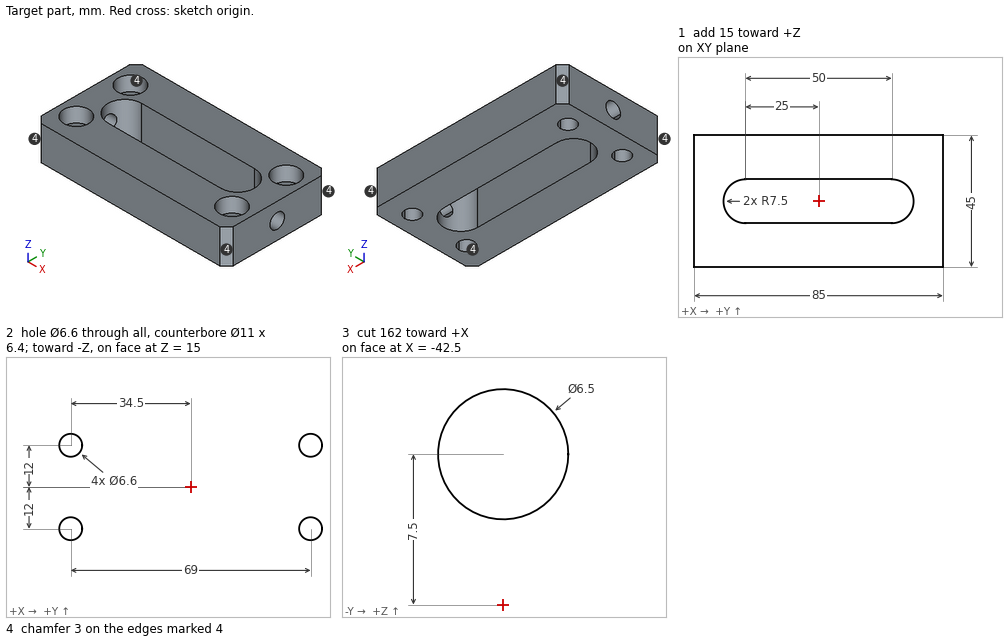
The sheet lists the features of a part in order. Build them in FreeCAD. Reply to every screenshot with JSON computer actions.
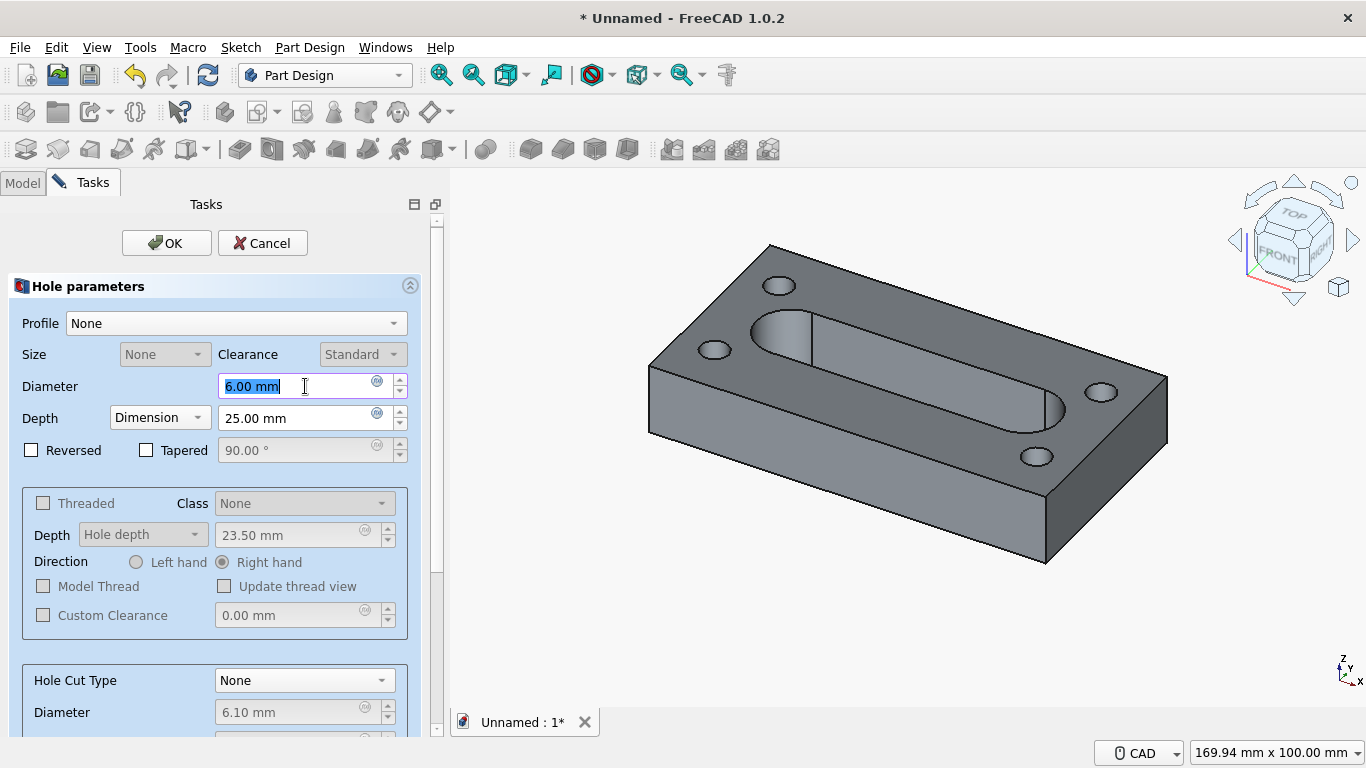
{"action": "type", "text": "6.6"}
{"action": "key", "text": "Tab"}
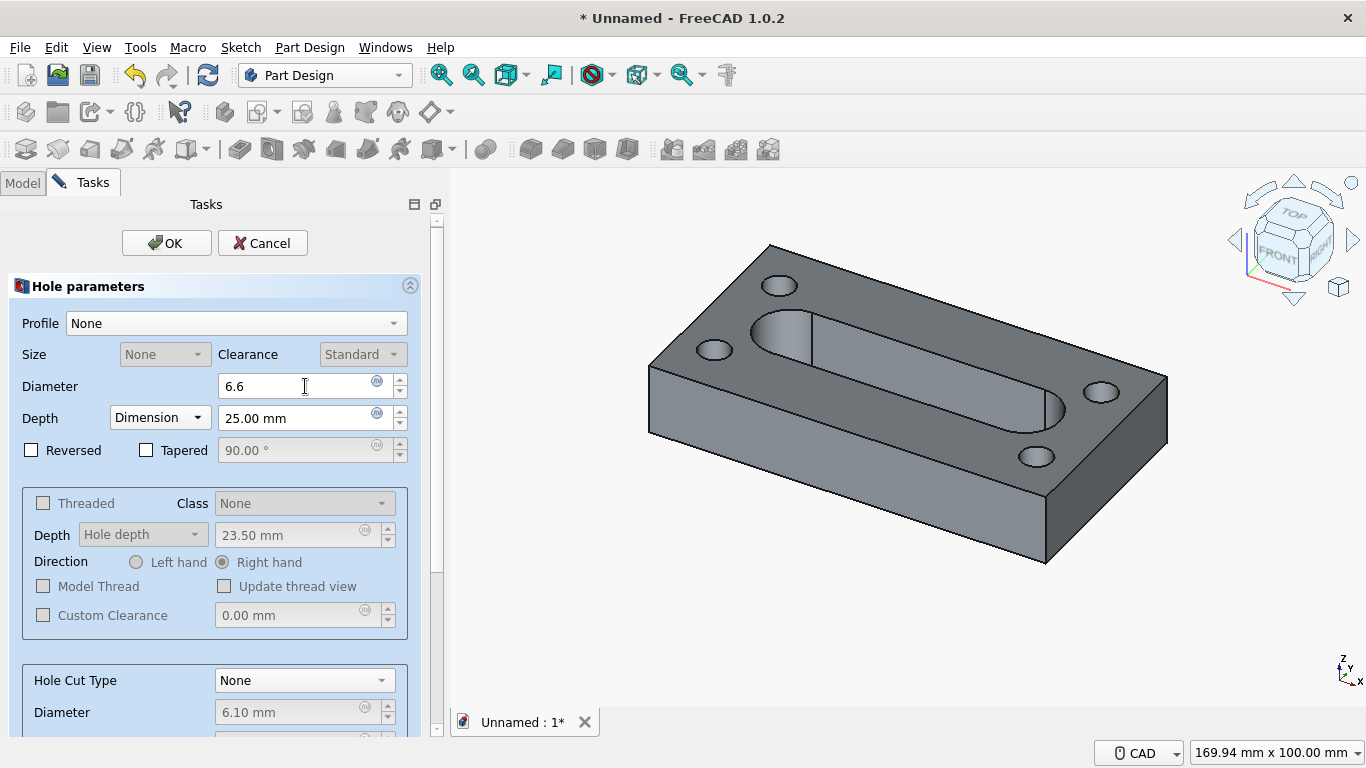
{"action": "left_click", "coordinate": [161, 418]}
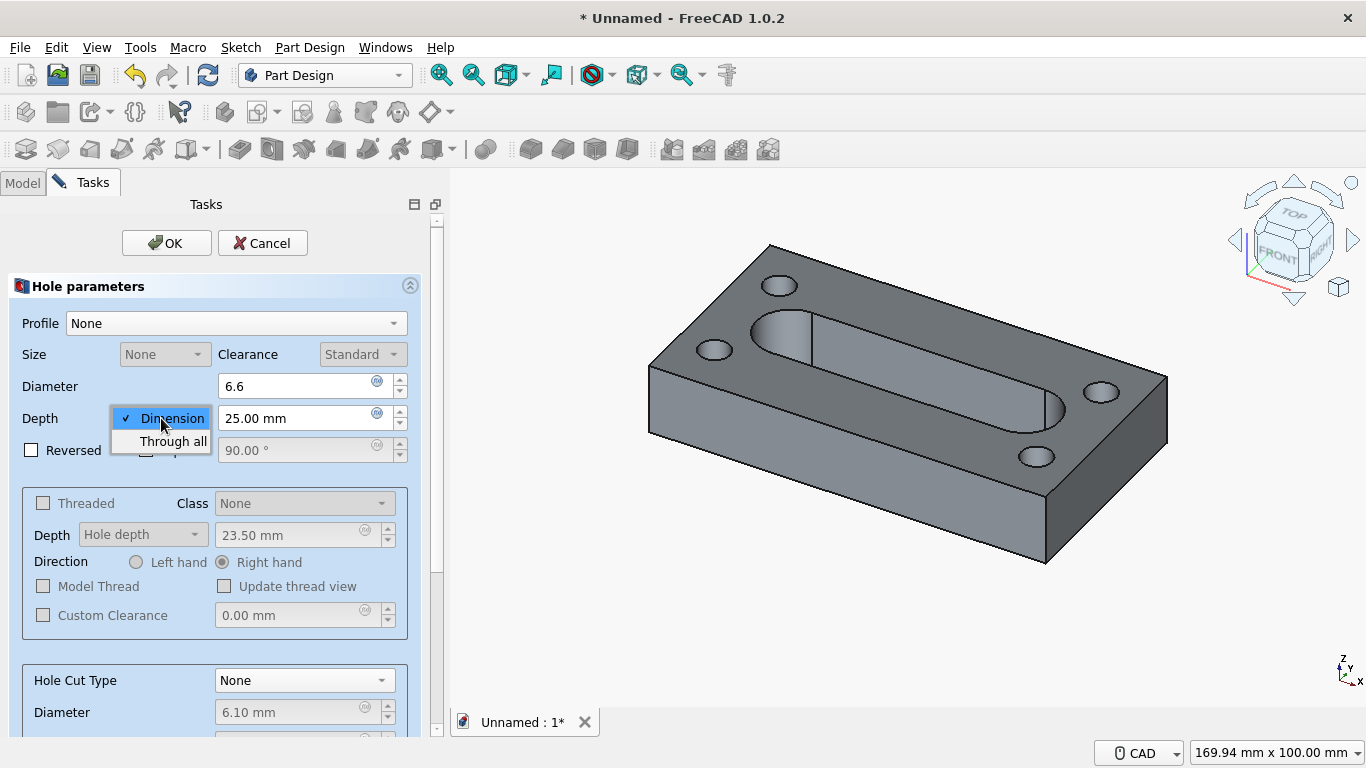
{"action": "left_click", "coordinate": [160, 442]}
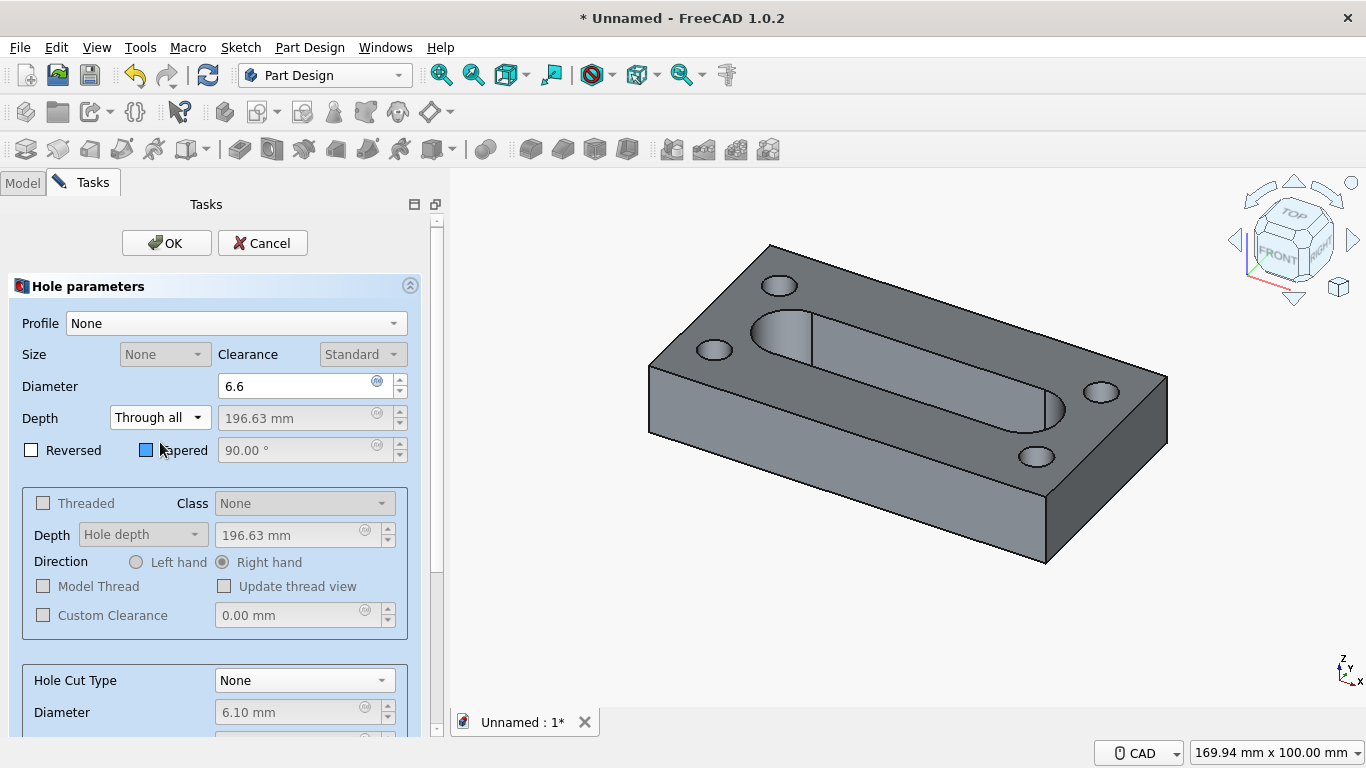
{"action": "left_click", "coordinate": [306, 680]}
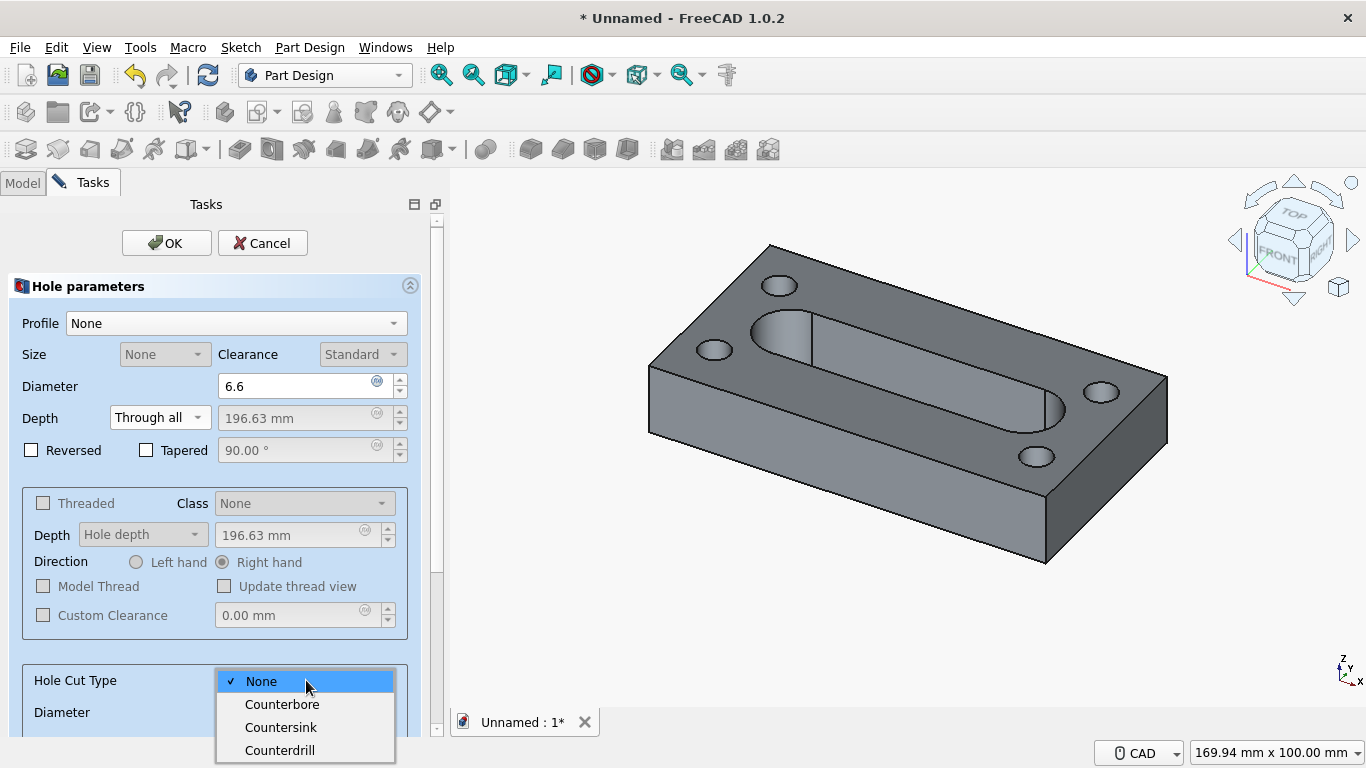
{"action": "left_click", "coordinate": [304, 704]}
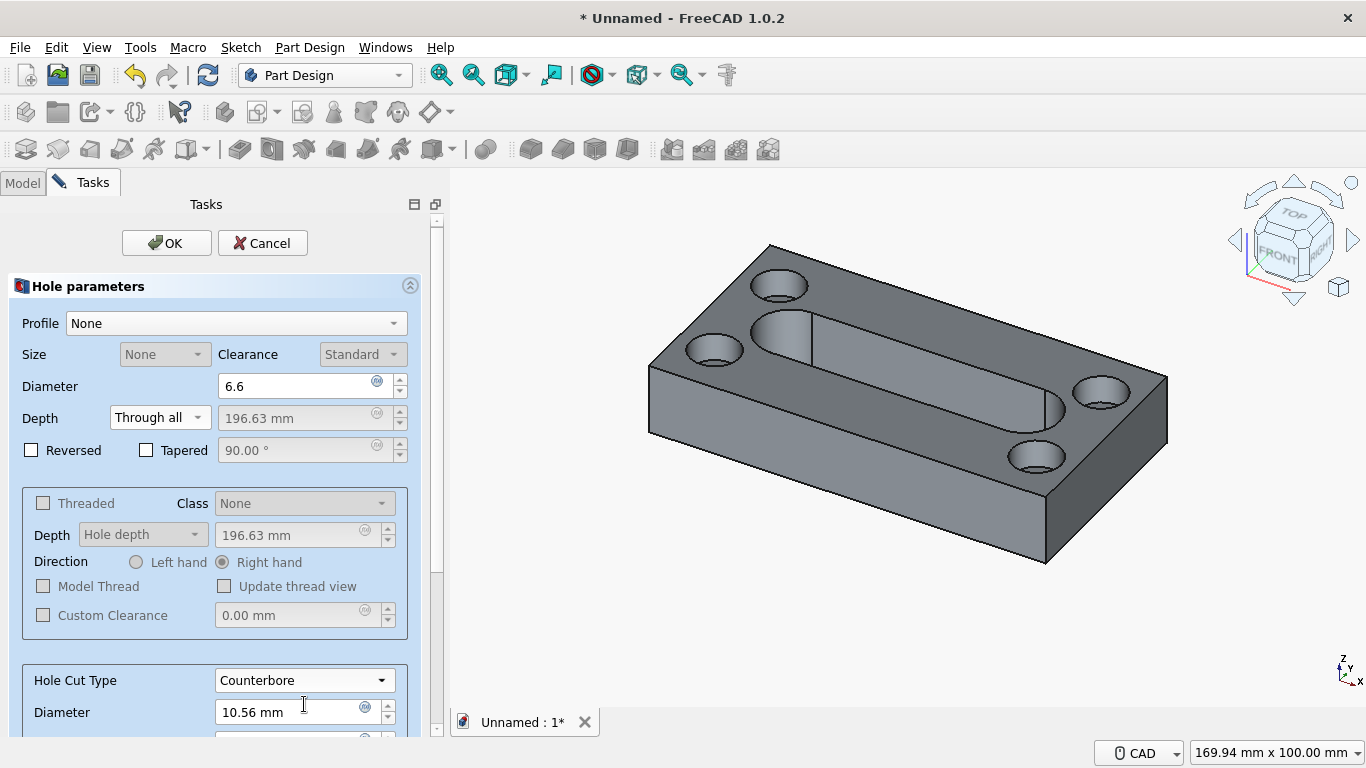
{"action": "triple_click", "coordinate": [298, 712]}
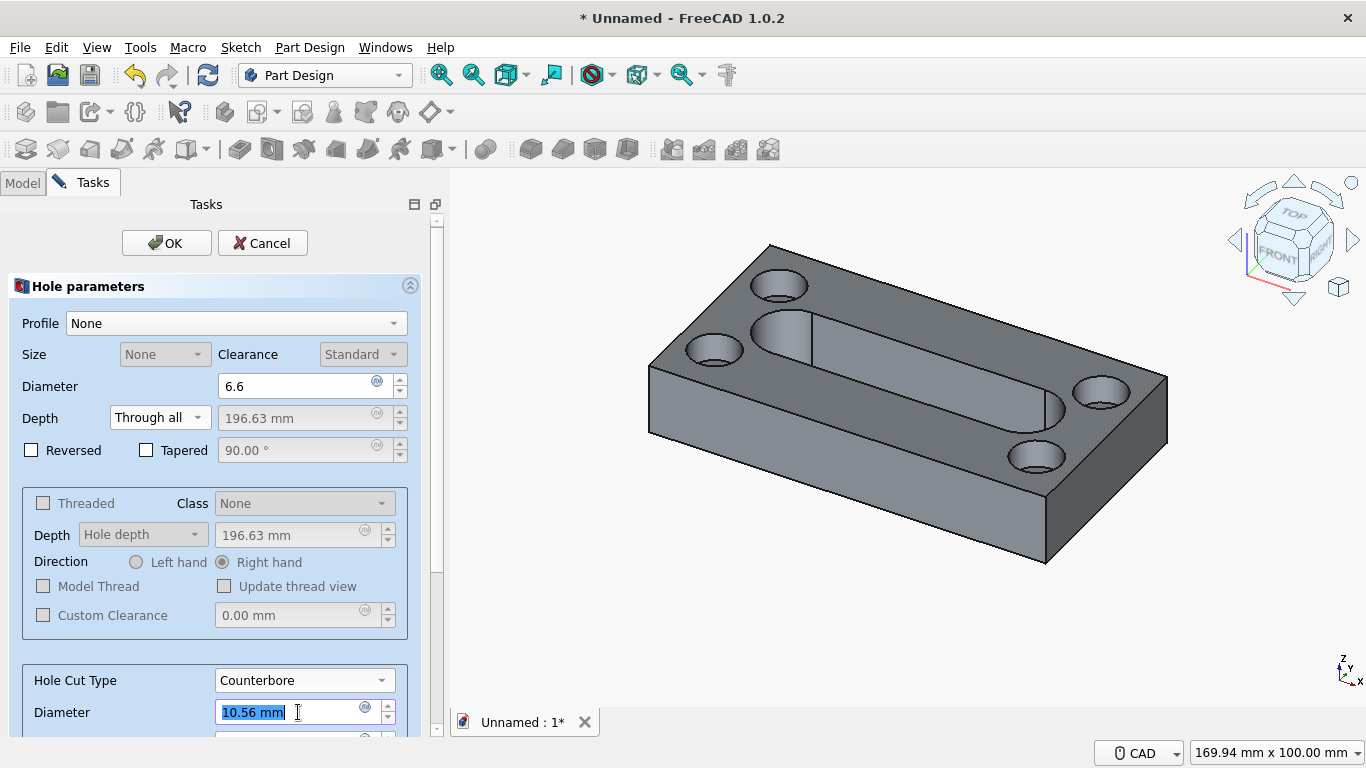
{"action": "type", "text": "11"}
{"action": "key", "text": "Tab"}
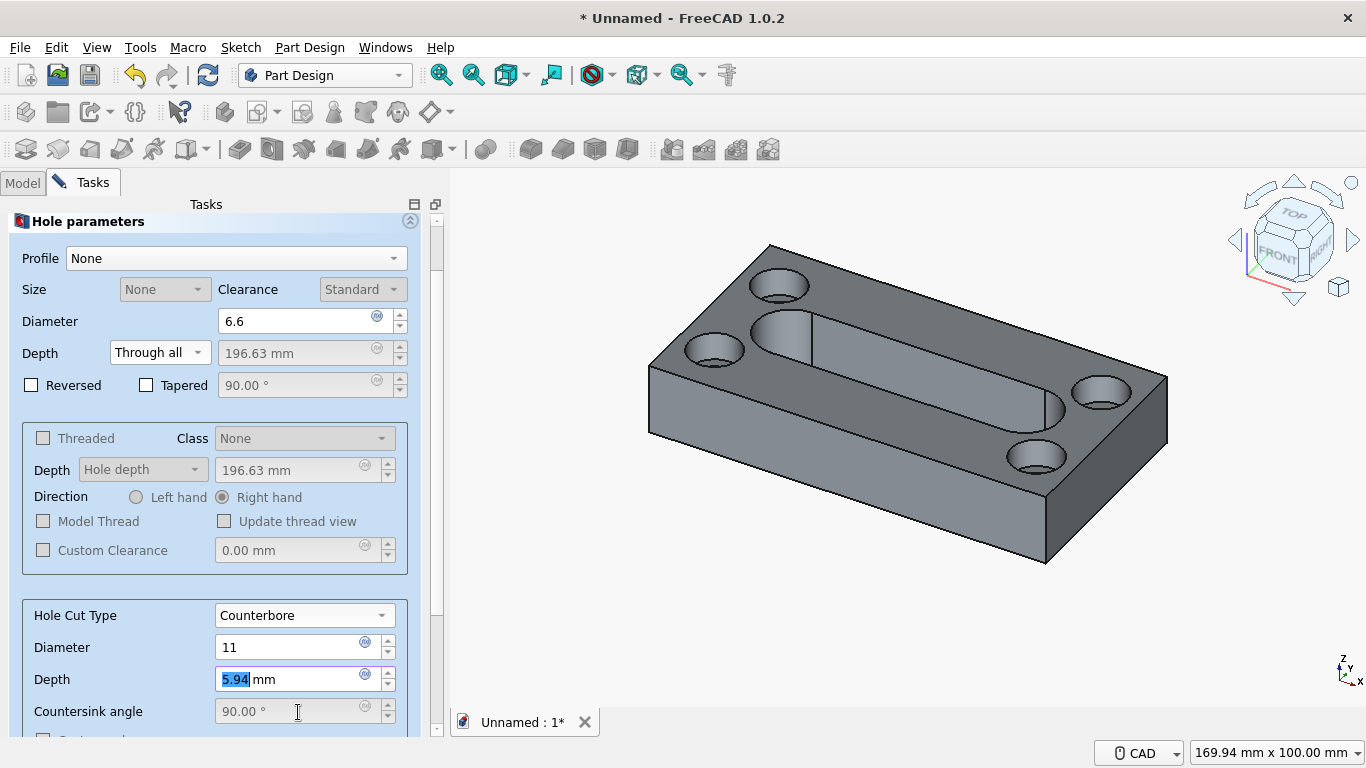
{"action": "type", "text": "6.4"}
{"action": "key", "text": "Tab"}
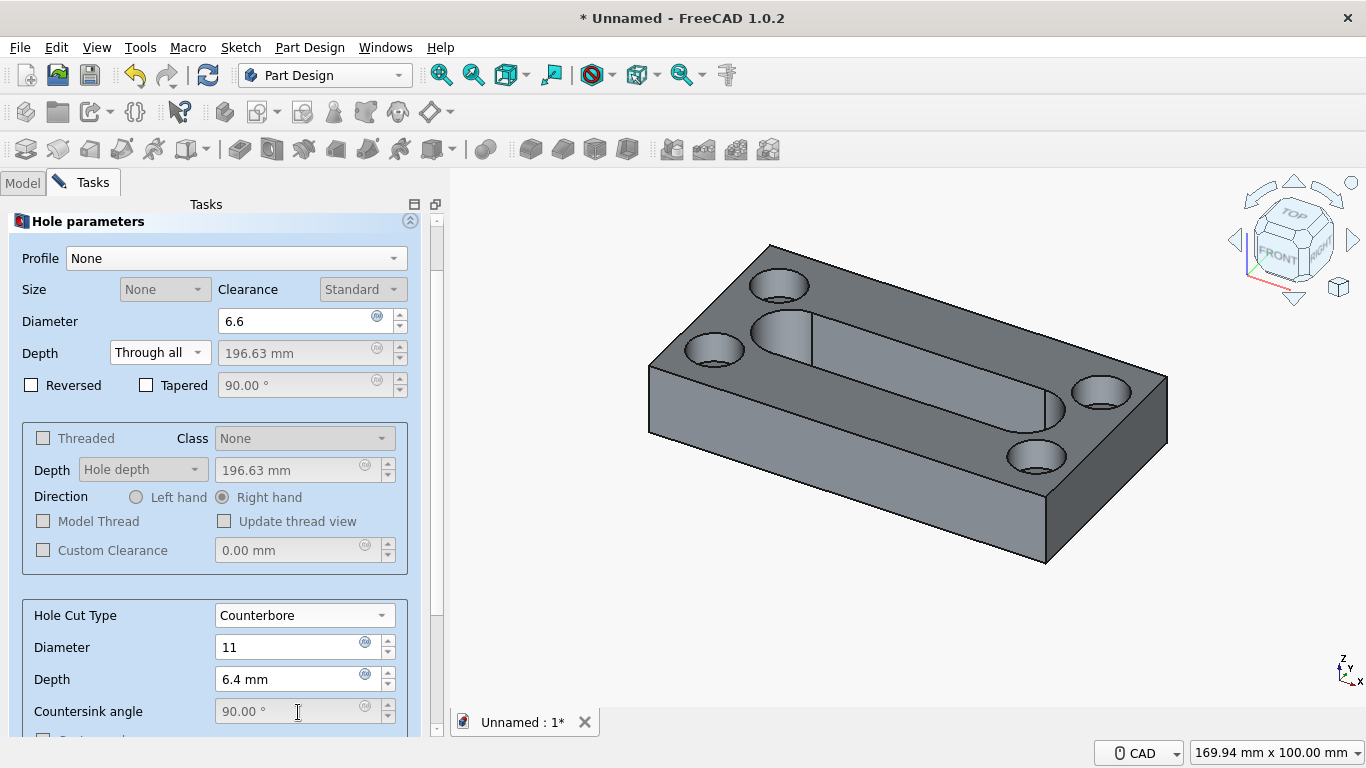
{"action": "scroll", "coordinate": [437, 475], "scroll_direction": "up", "scroll_amount": 2}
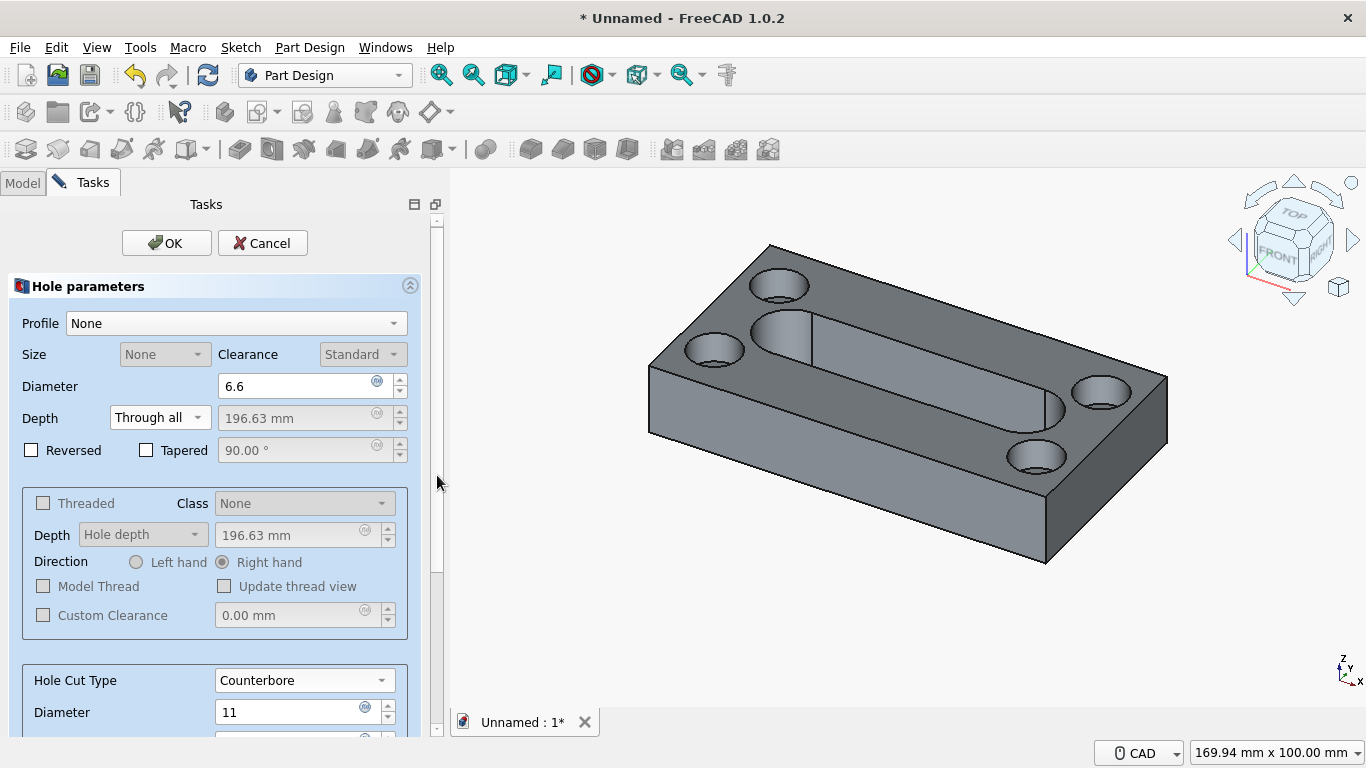
{"action": "left_click", "coordinate": [167, 243]}